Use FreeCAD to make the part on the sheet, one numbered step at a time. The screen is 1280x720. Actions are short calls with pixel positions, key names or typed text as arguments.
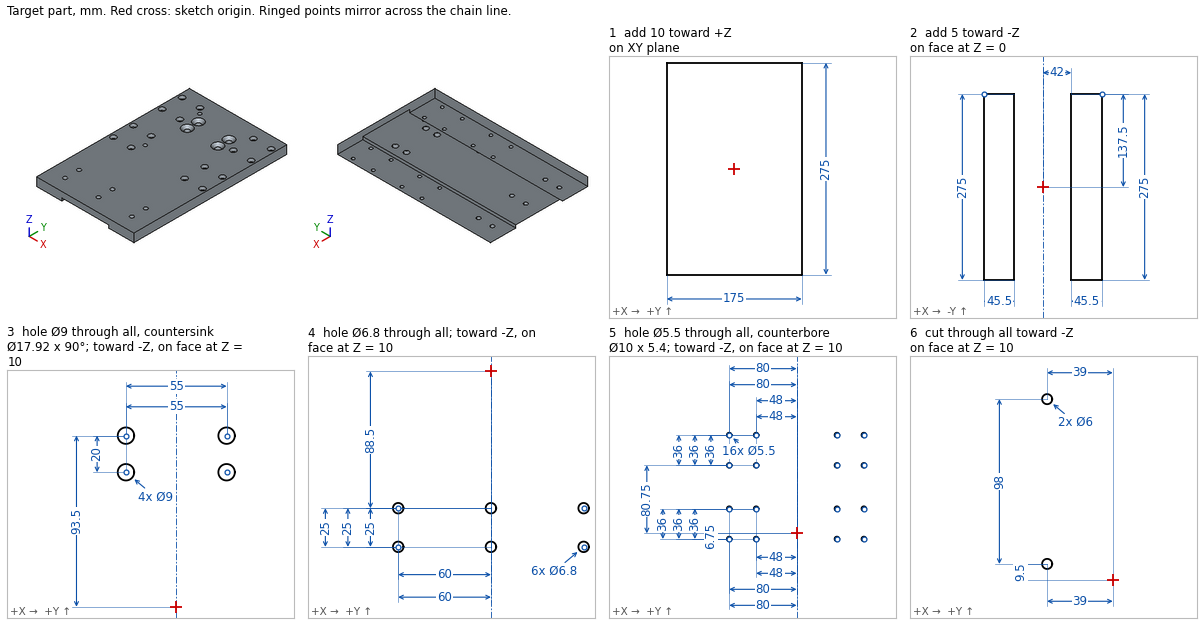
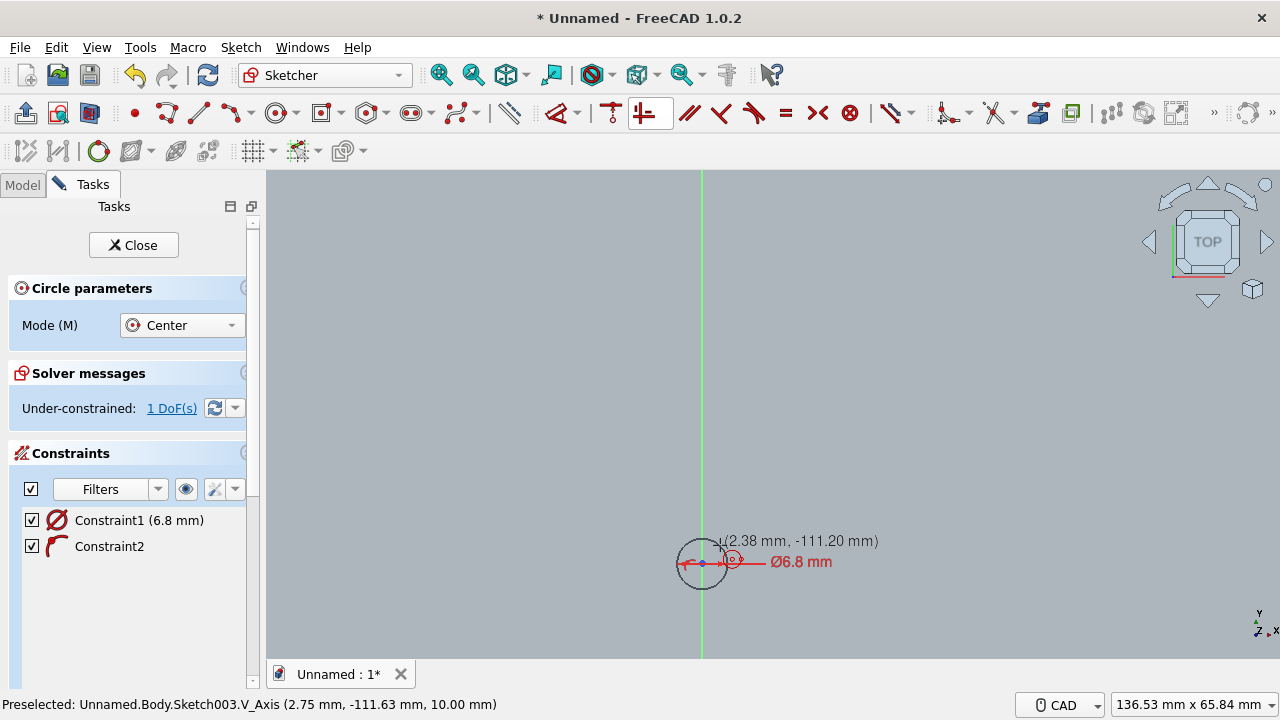
scroll(706, 566, down, 5)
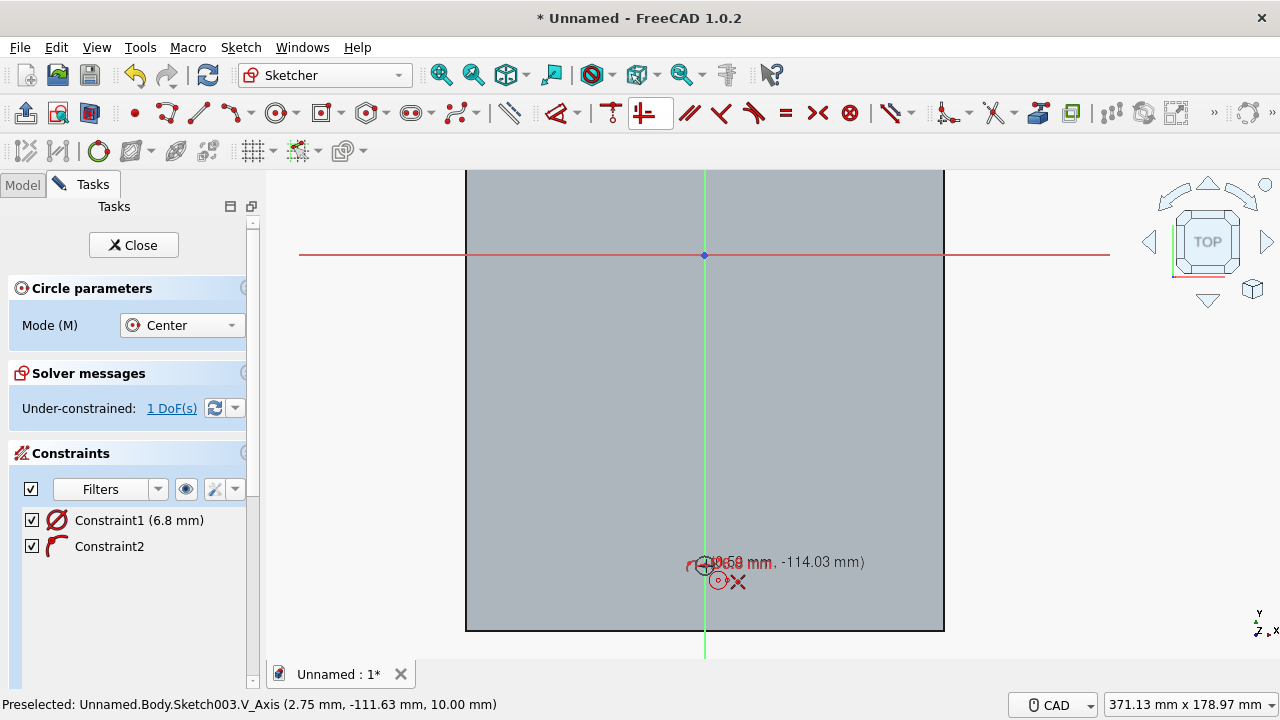
scroll(541, 565, up, 5)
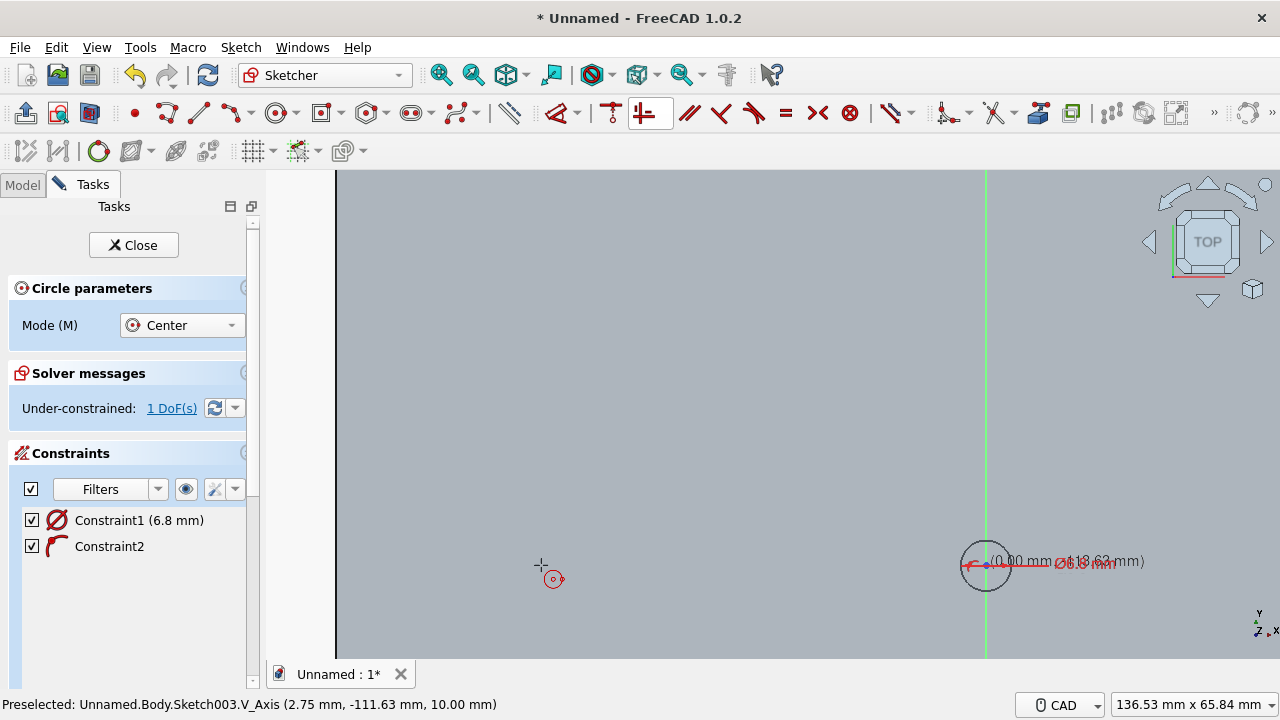
click(541, 565)
move(558, 547)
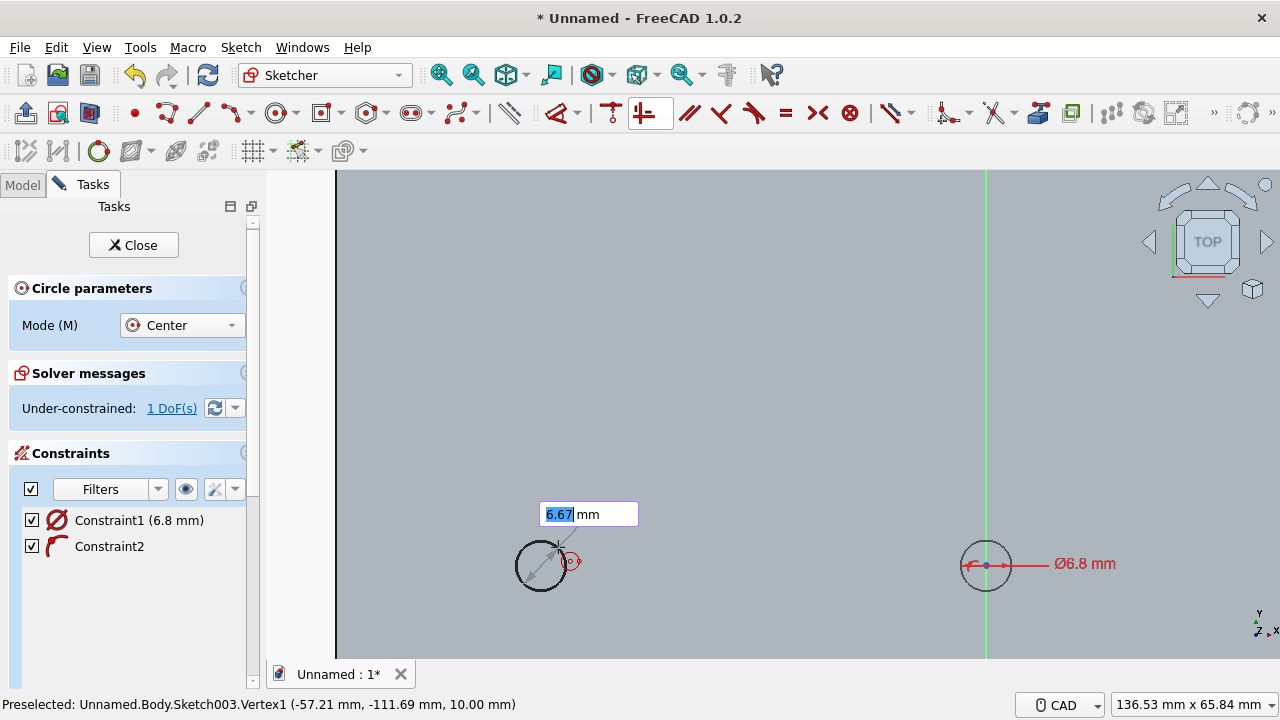
text(6.8)
key(Return)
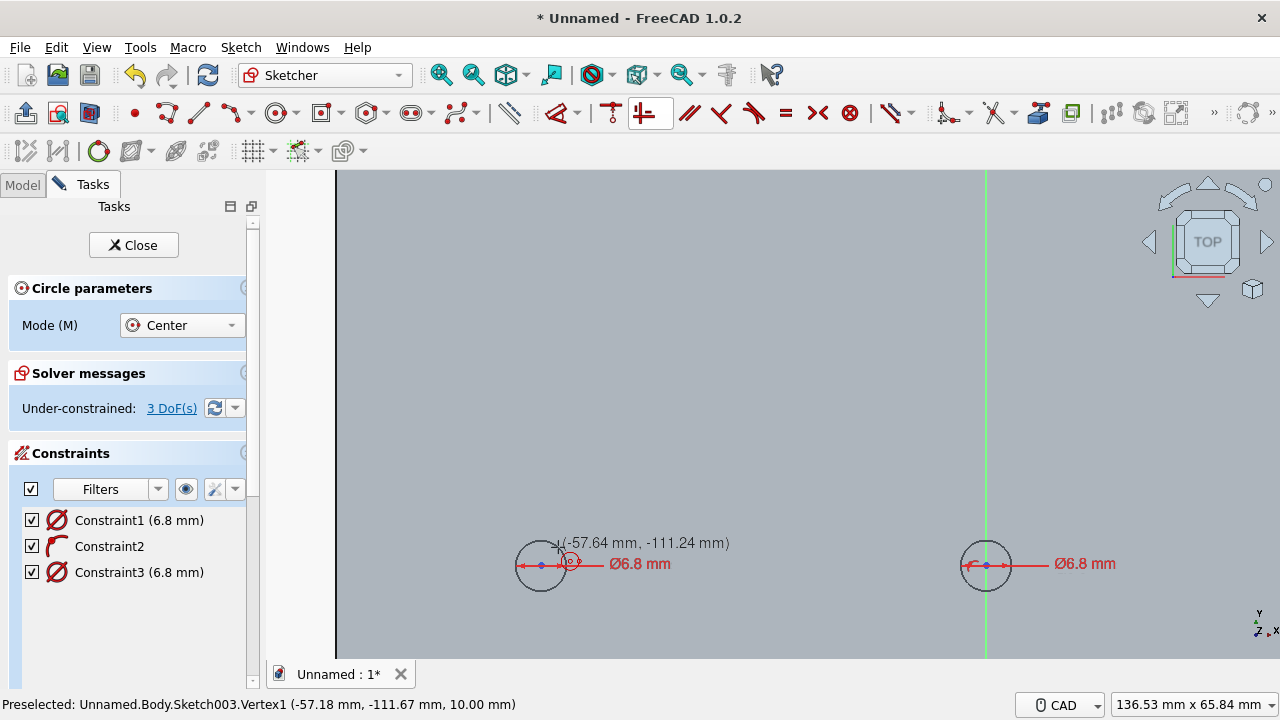
scroll(541, 565, down, 5)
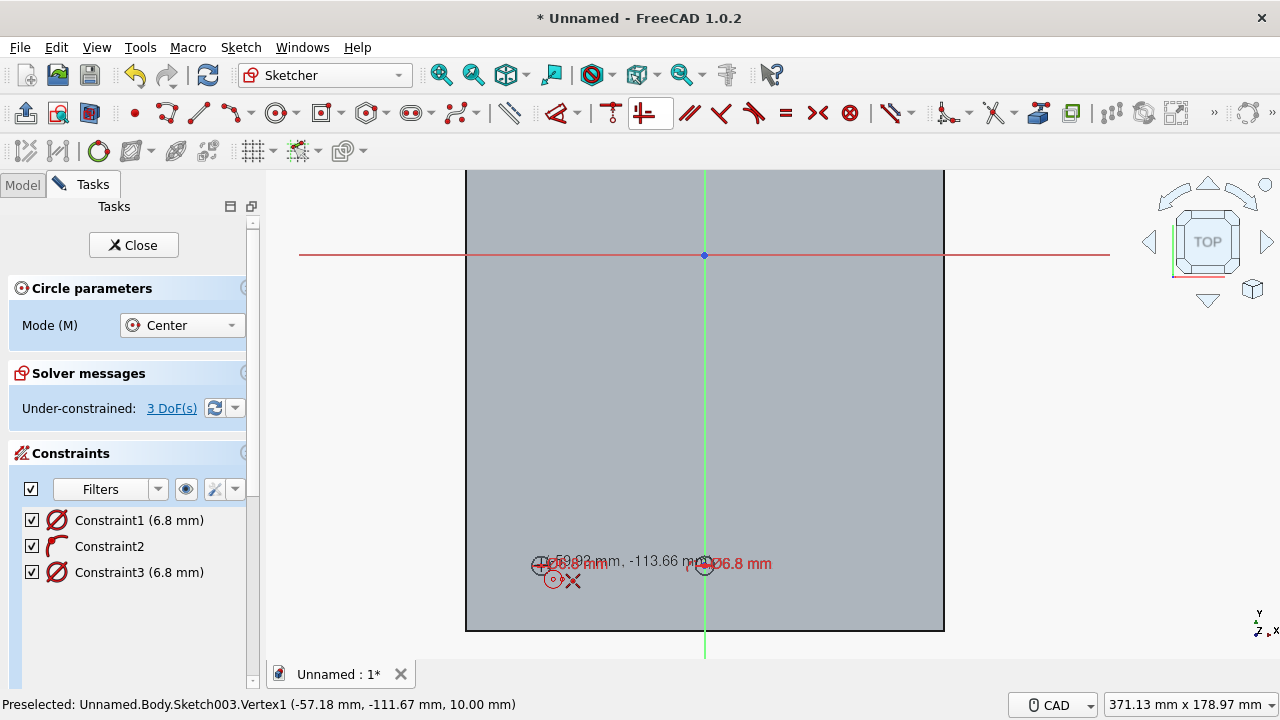
scroll(869, 565, up, 5)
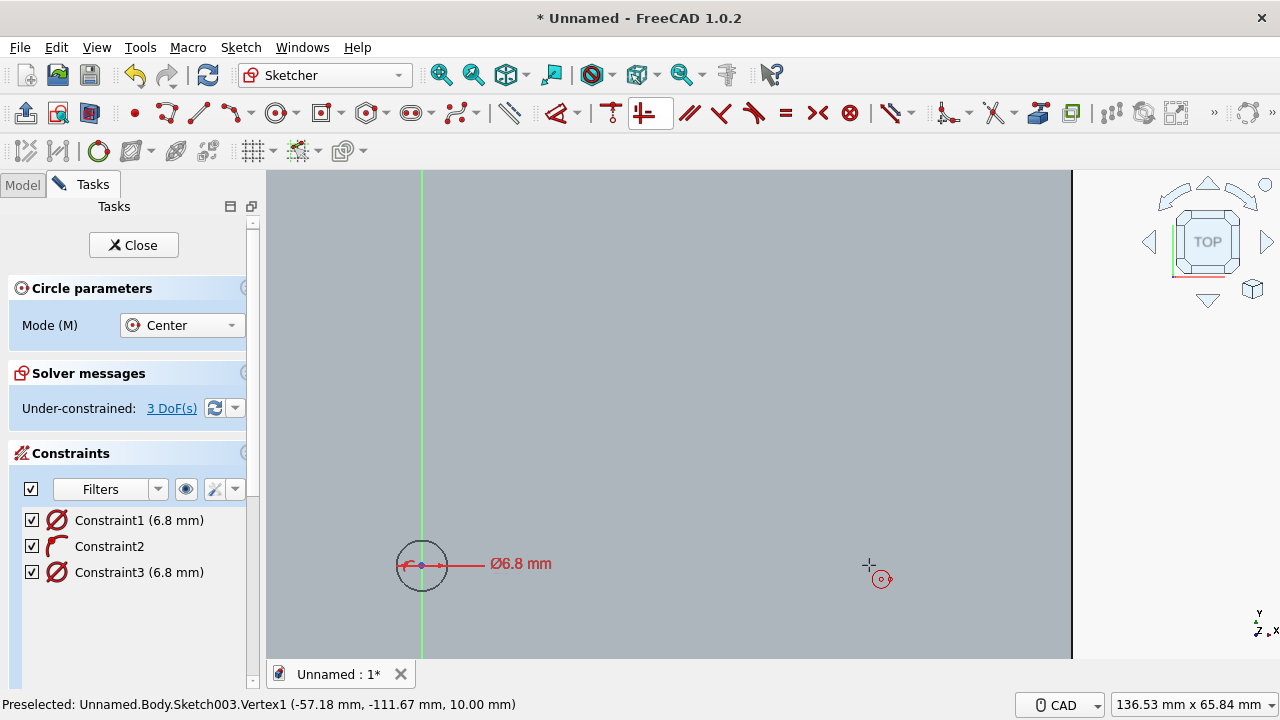
click(868, 565)
move(885, 547)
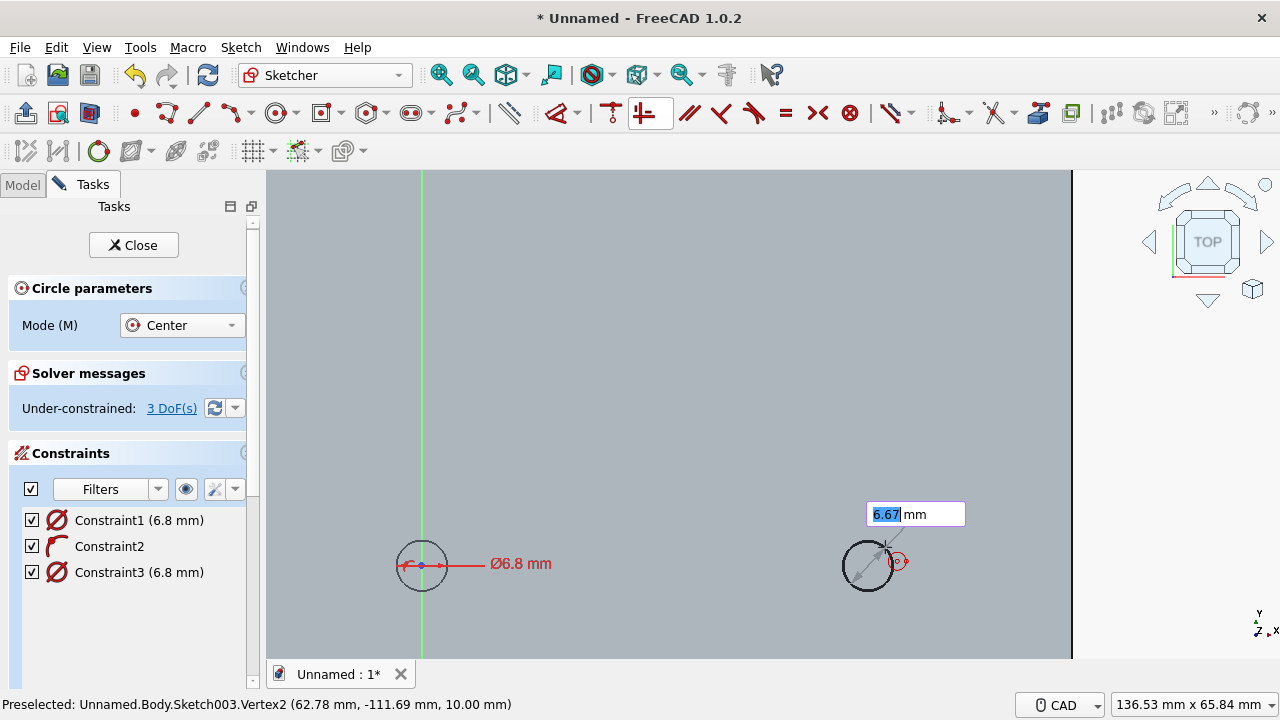
text(6.8)
key(Return)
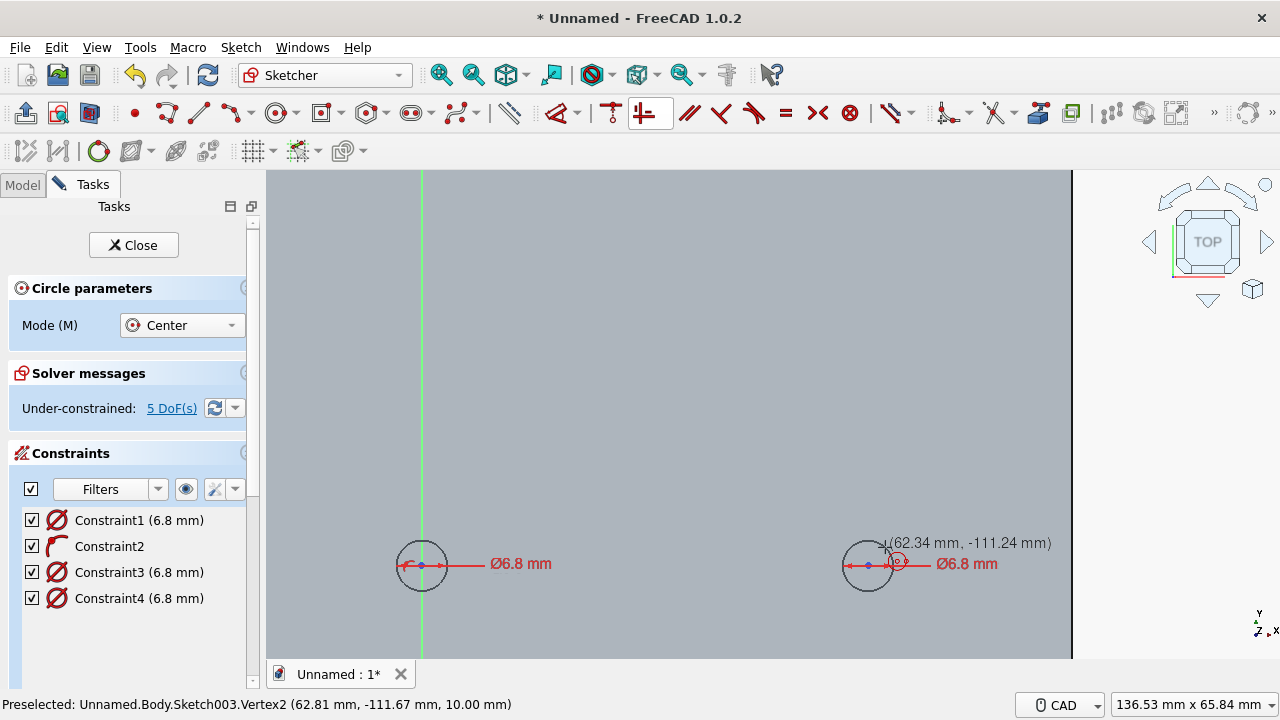
click(422, 379)
move(440, 361)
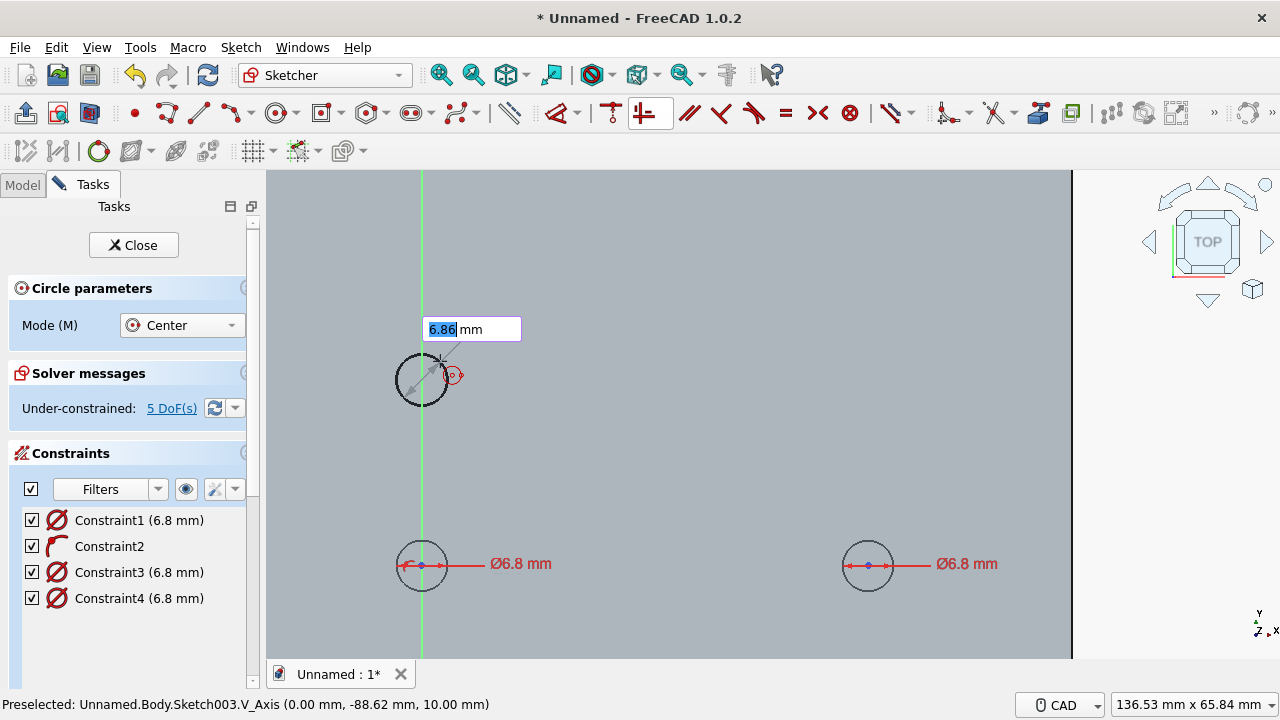
text(6.8)
key(Return)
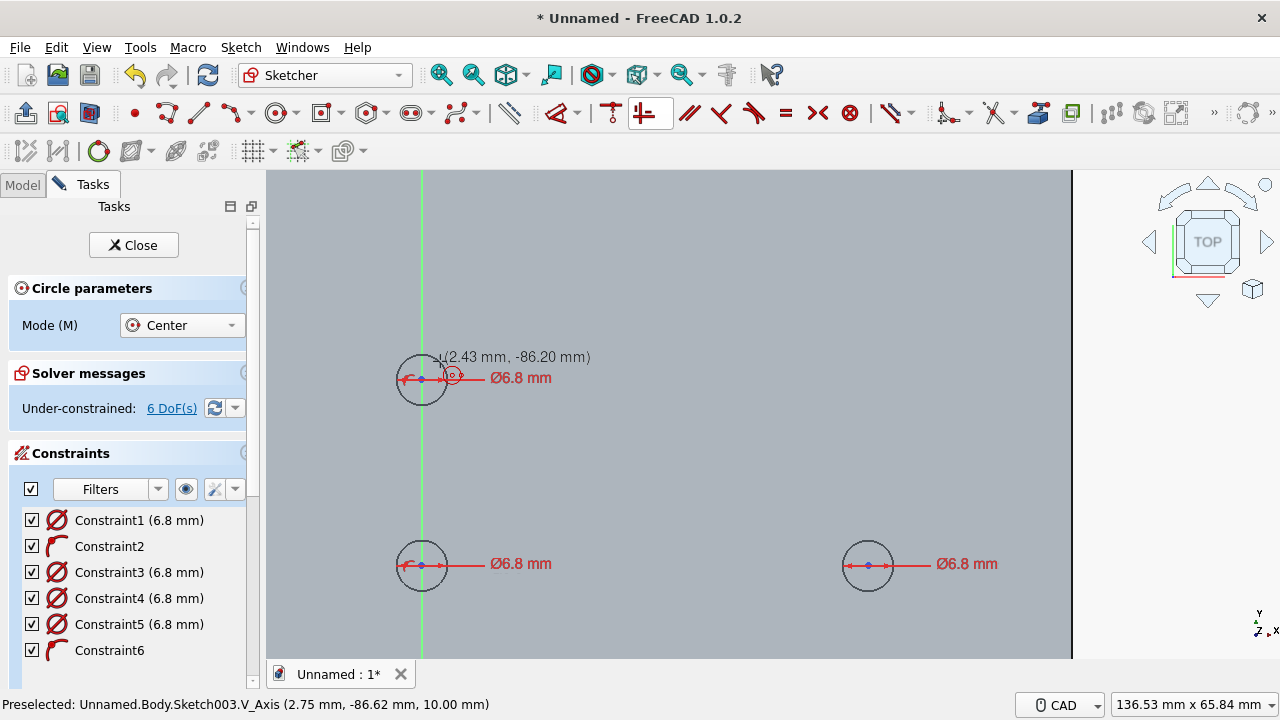
scroll(869, 565, down, 5)